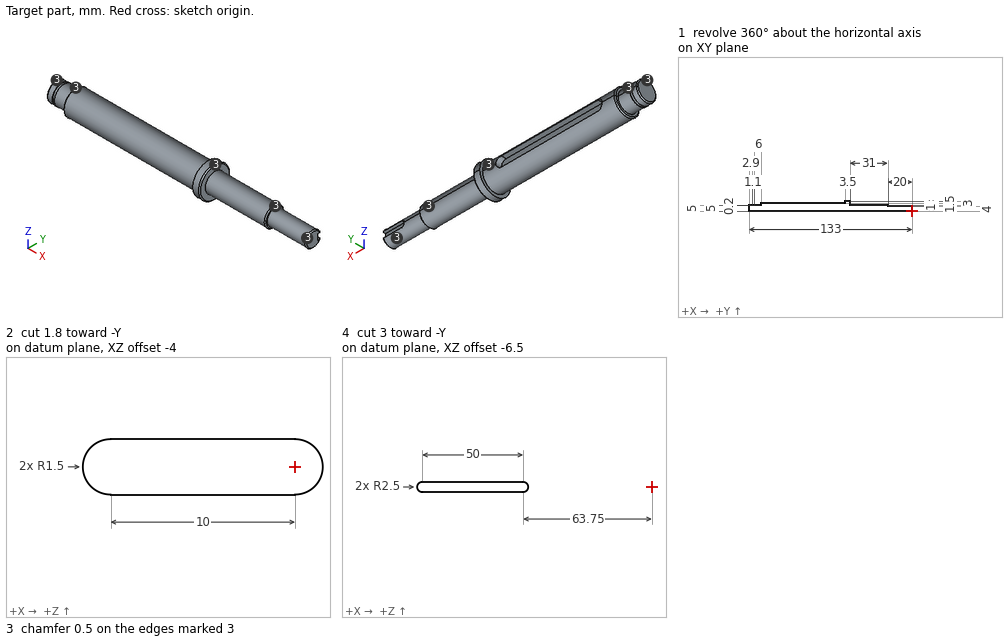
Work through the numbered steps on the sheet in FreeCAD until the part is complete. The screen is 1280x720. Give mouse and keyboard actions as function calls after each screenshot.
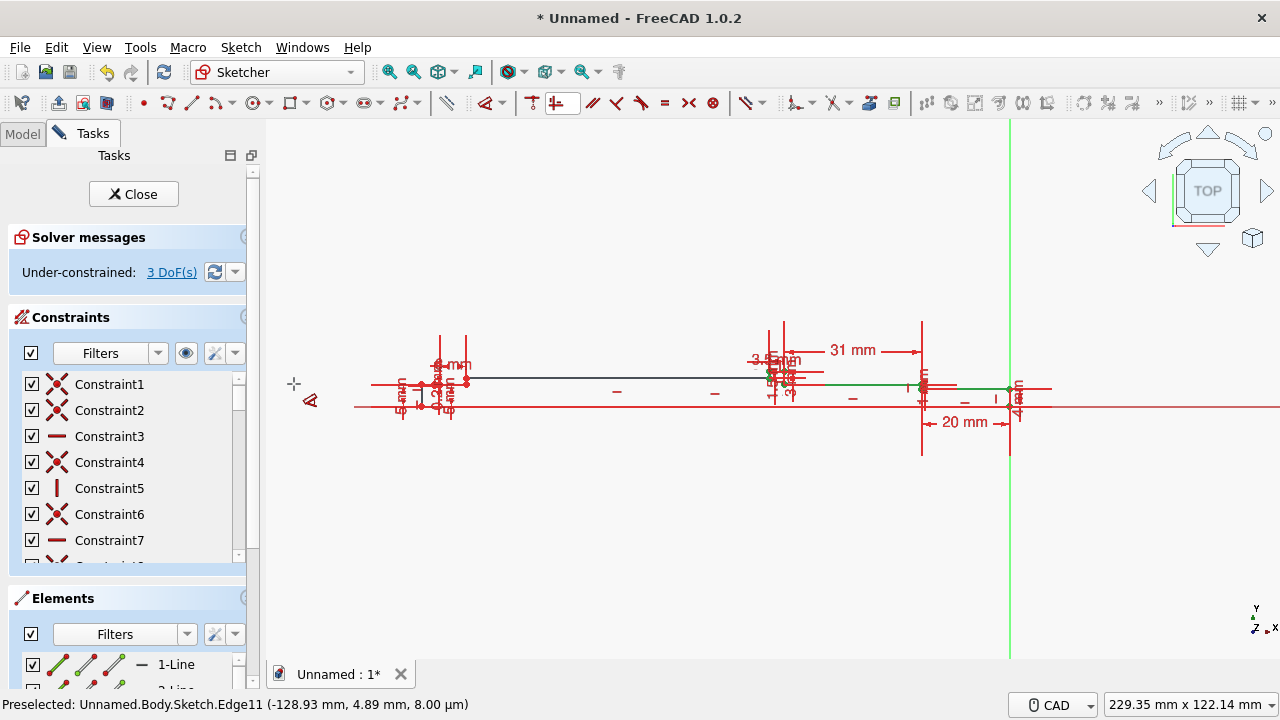
scroll(438, 386, up, 12)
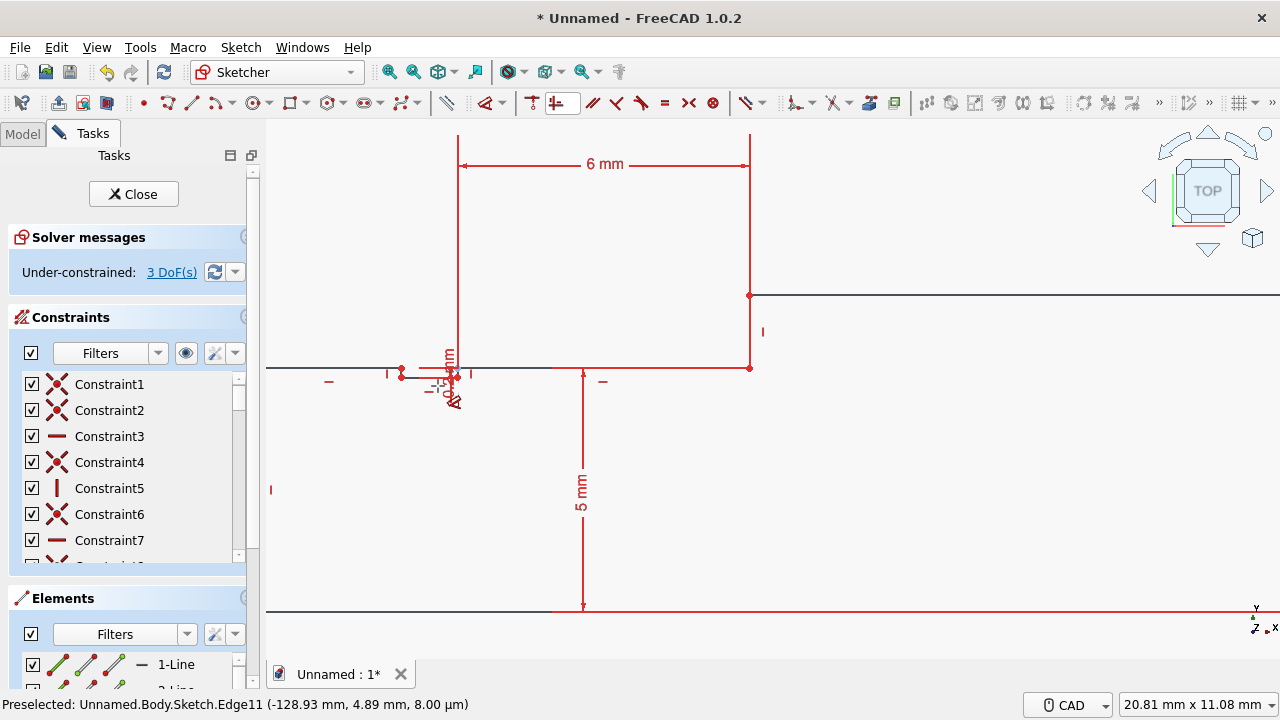
click(441, 378)
click(430, 344)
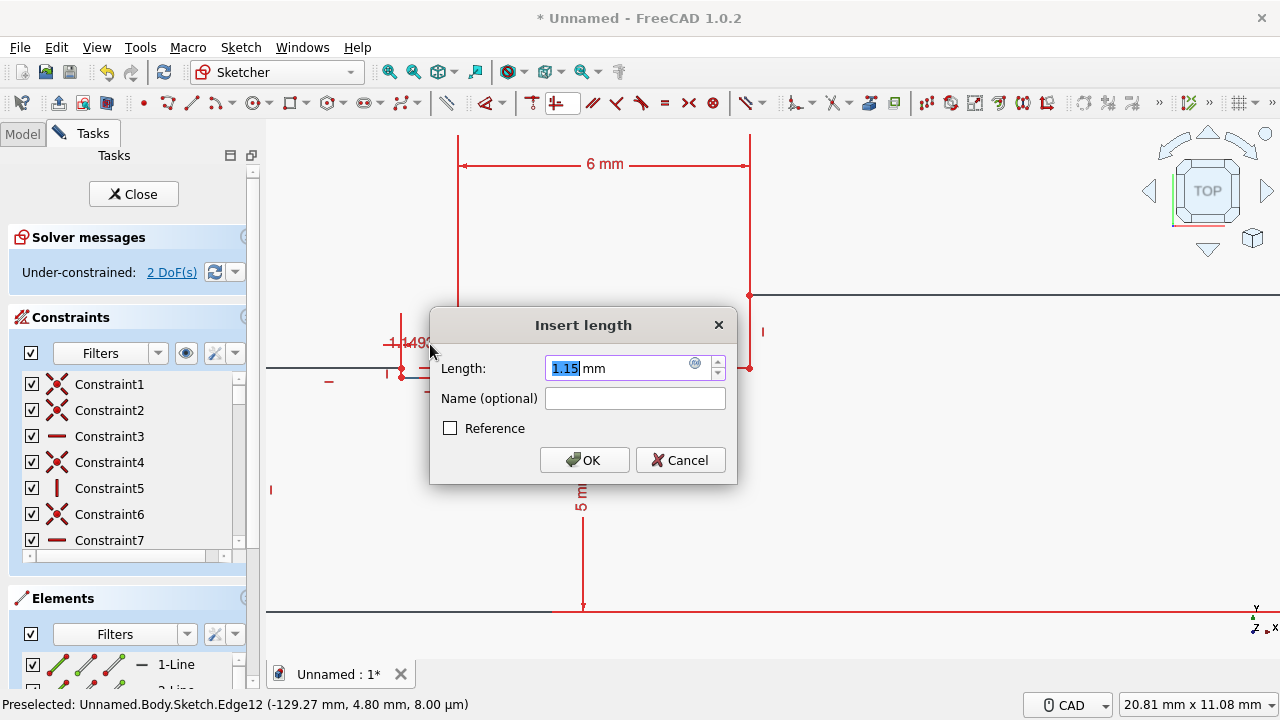
text(1.1)
key(Return)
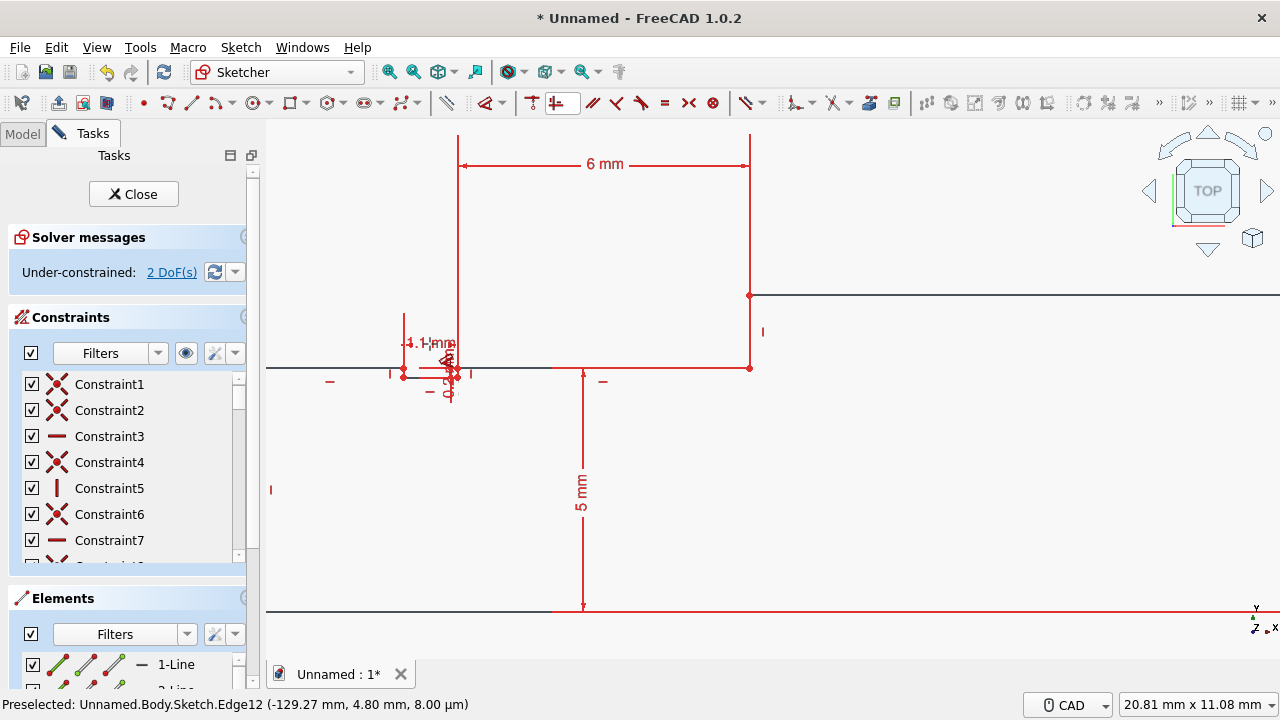
scroll(426, 386, down, 12)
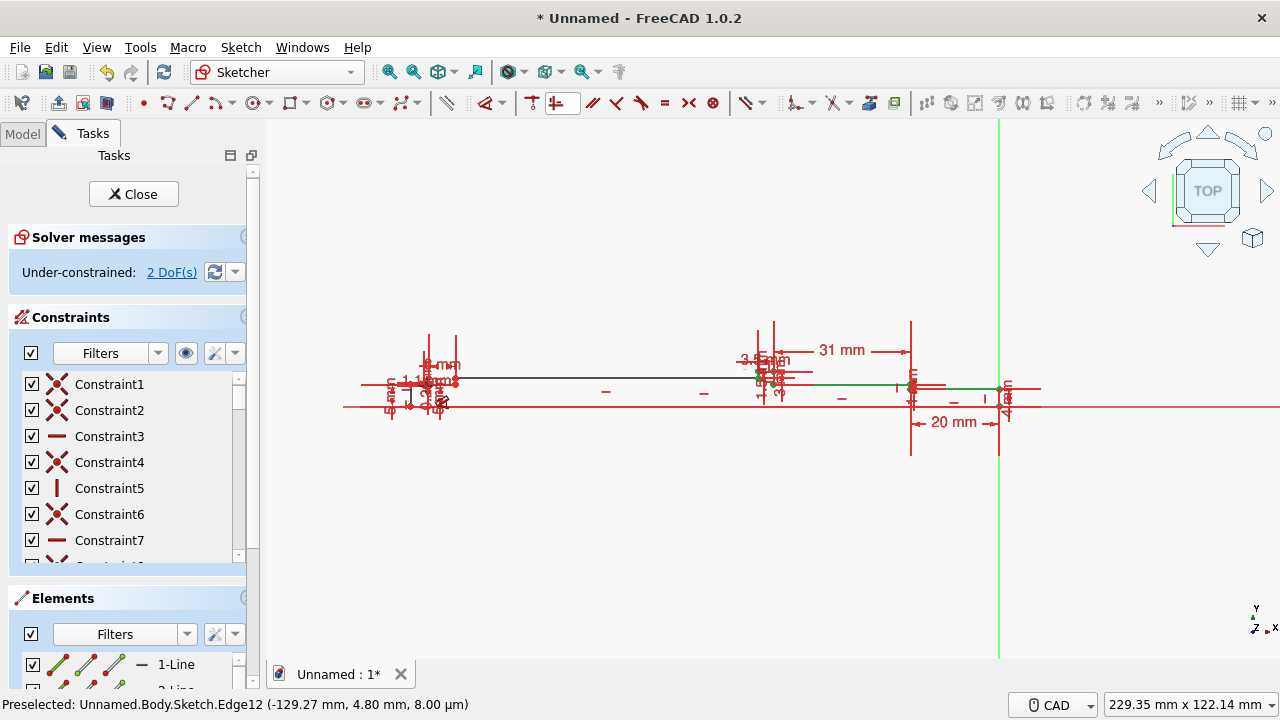
scroll(420, 385, up, 7)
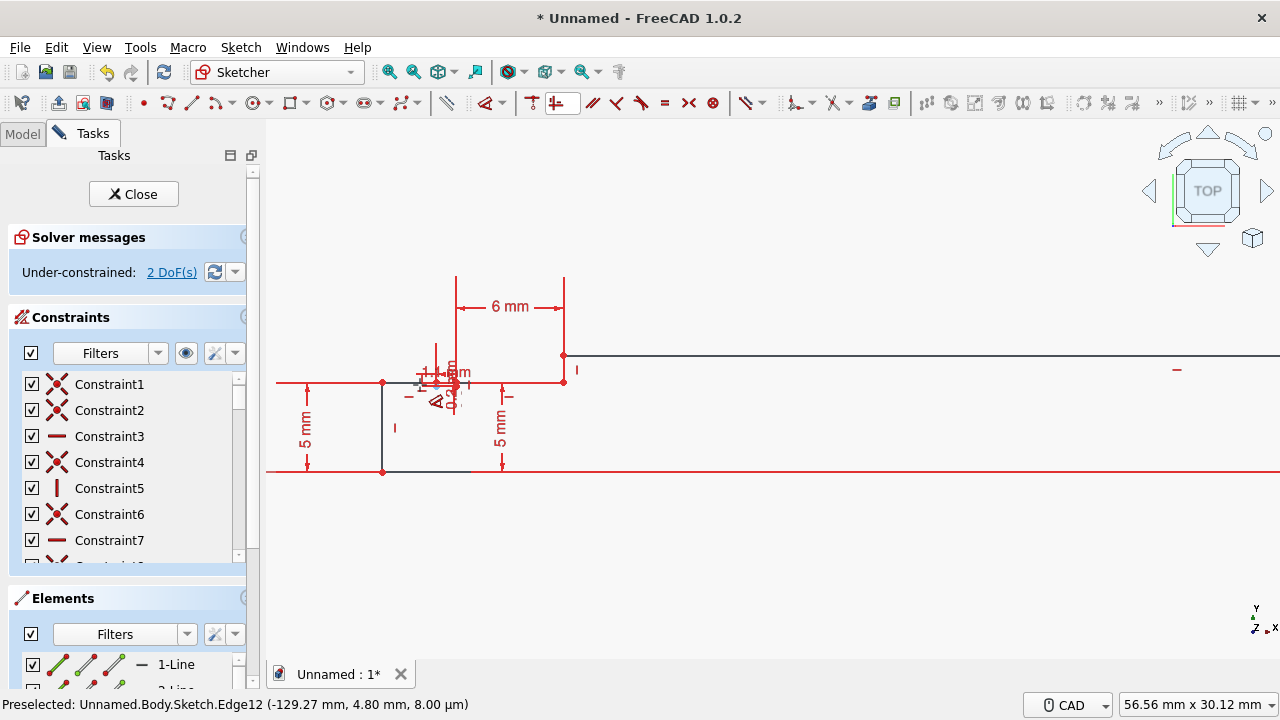
click(420, 383)
click(409, 349)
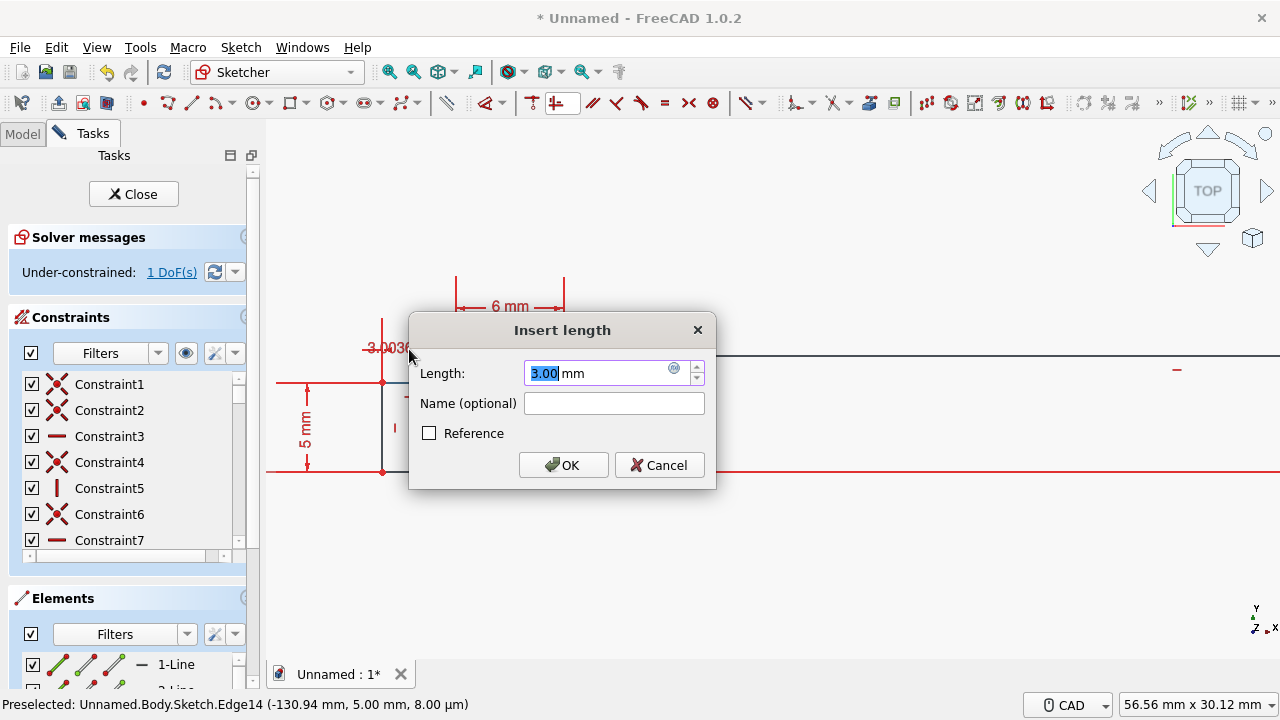
text(2.9)
key(Return)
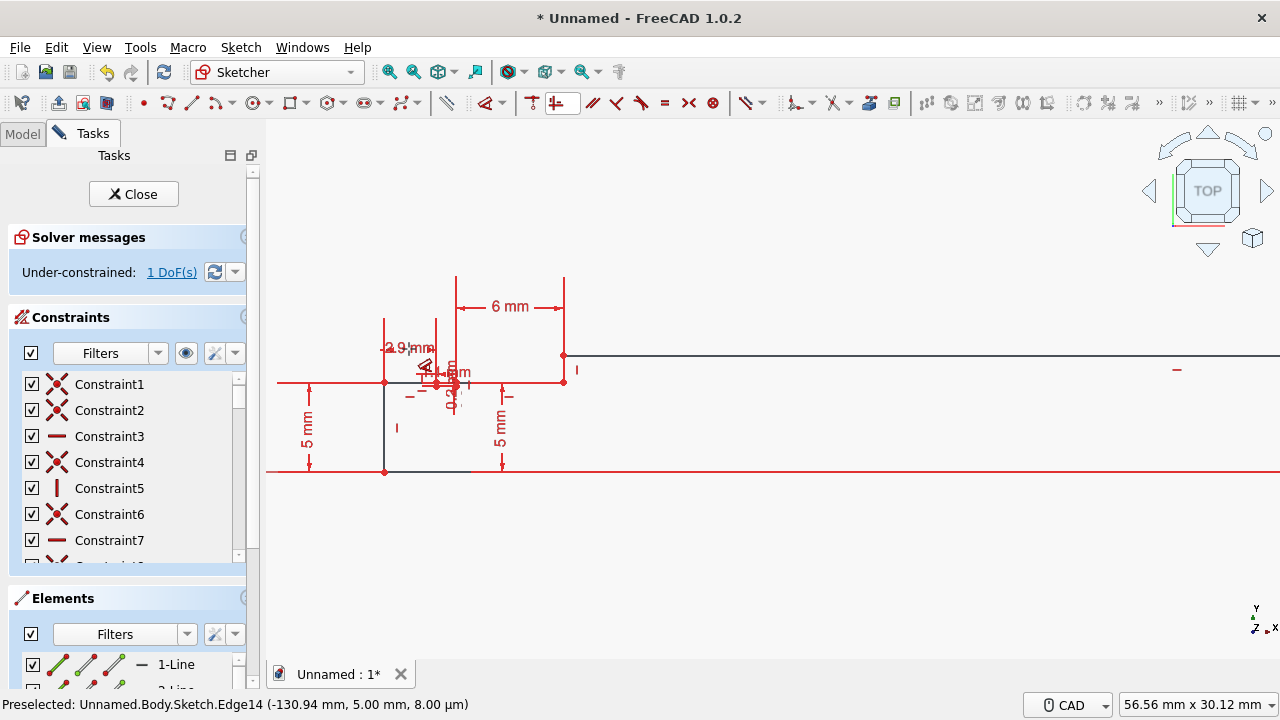
scroll(419, 385, down, 7)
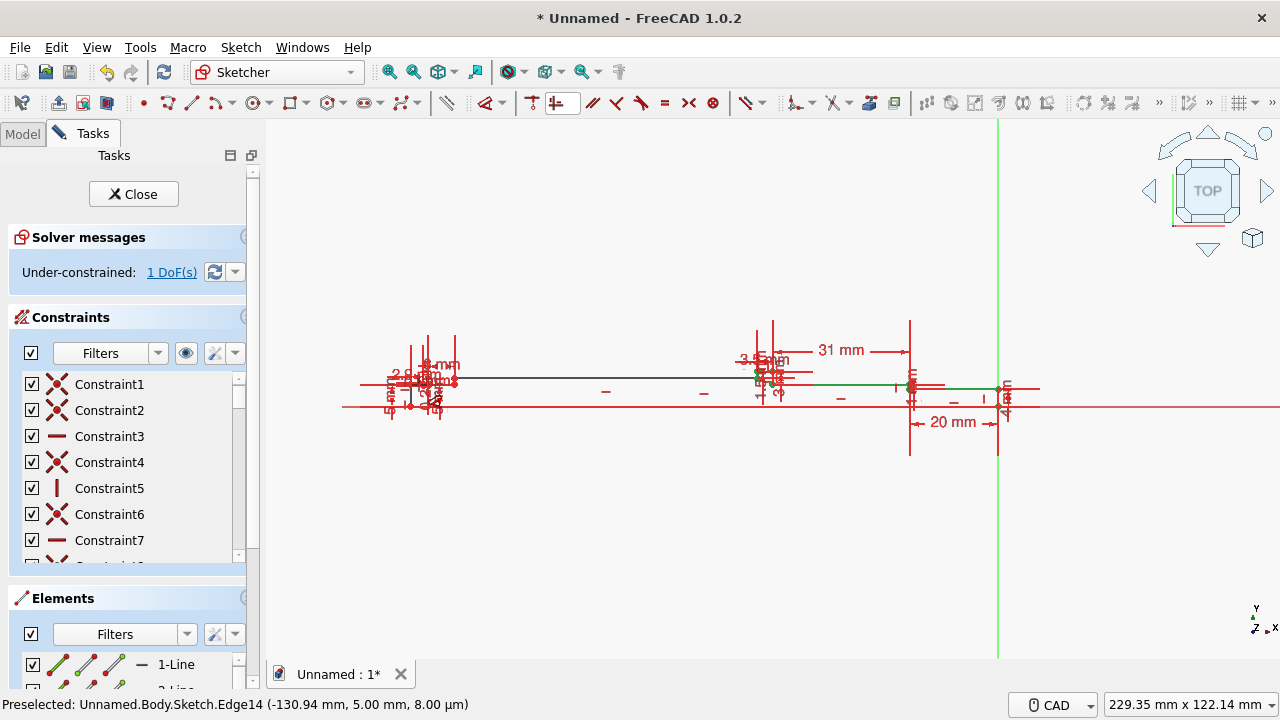
click(587, 407)
click(704, 441)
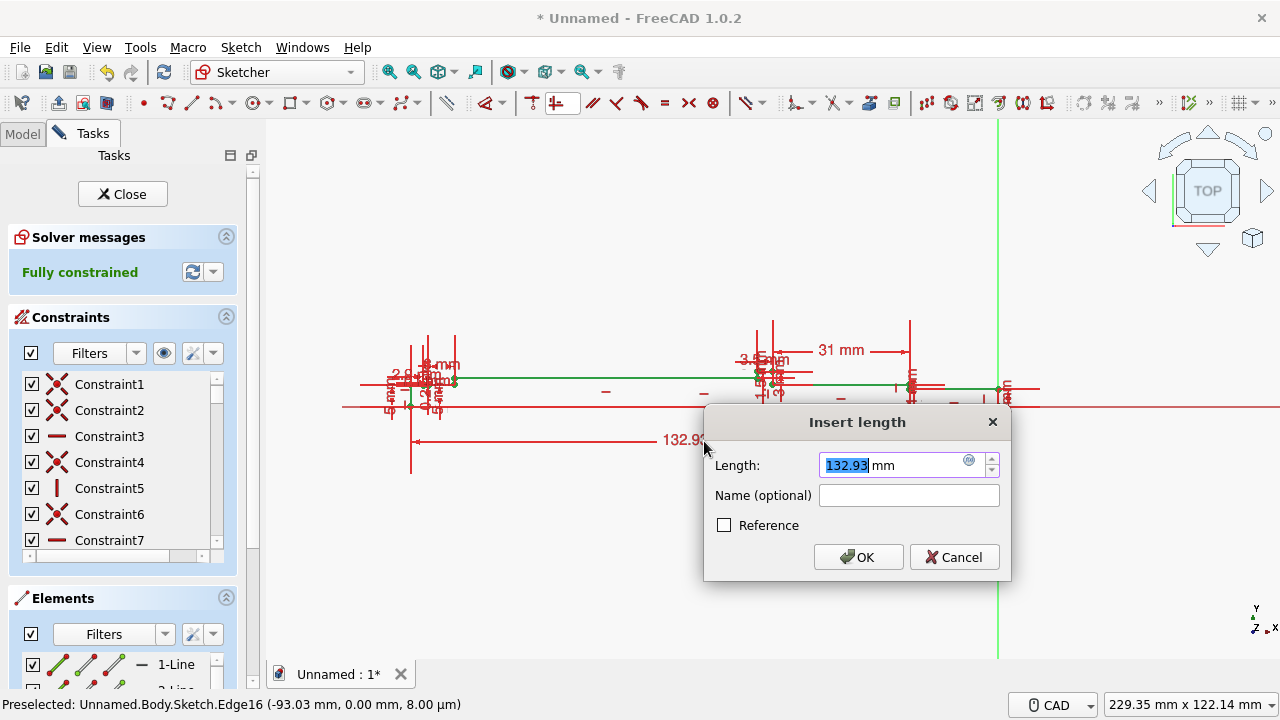
text(133)
key(Return)
key(Escape)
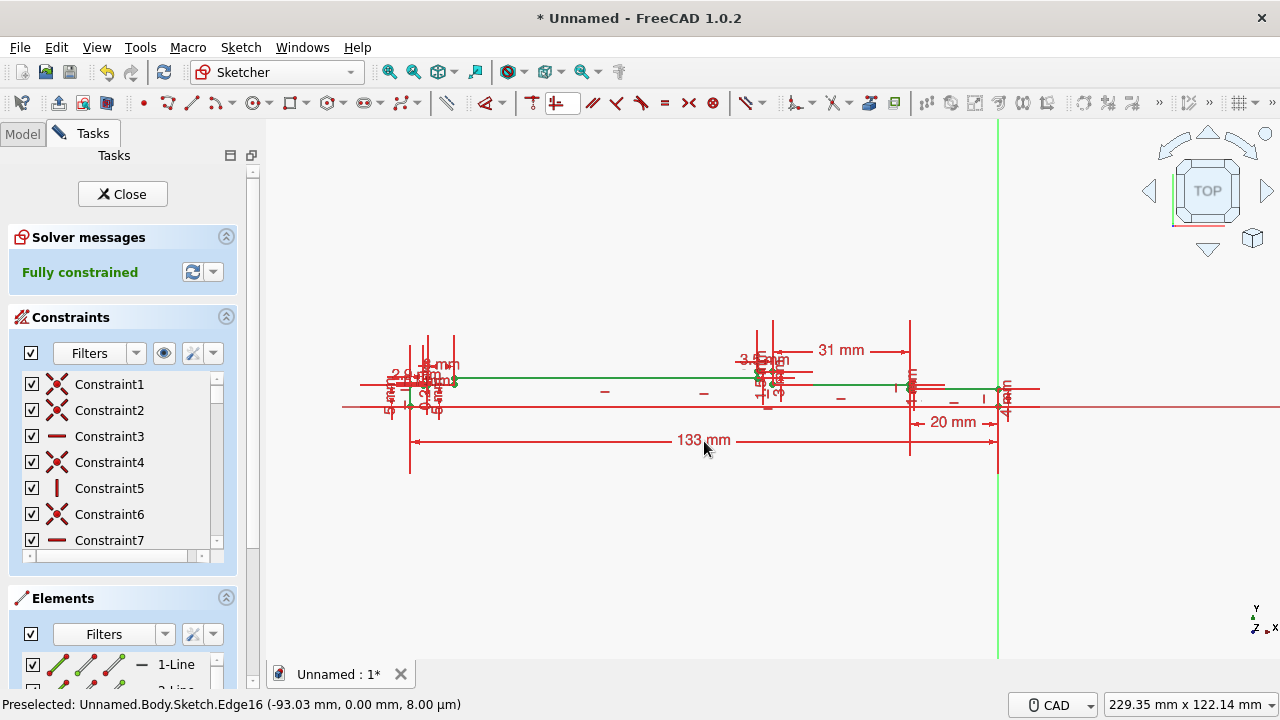
click(123, 194)